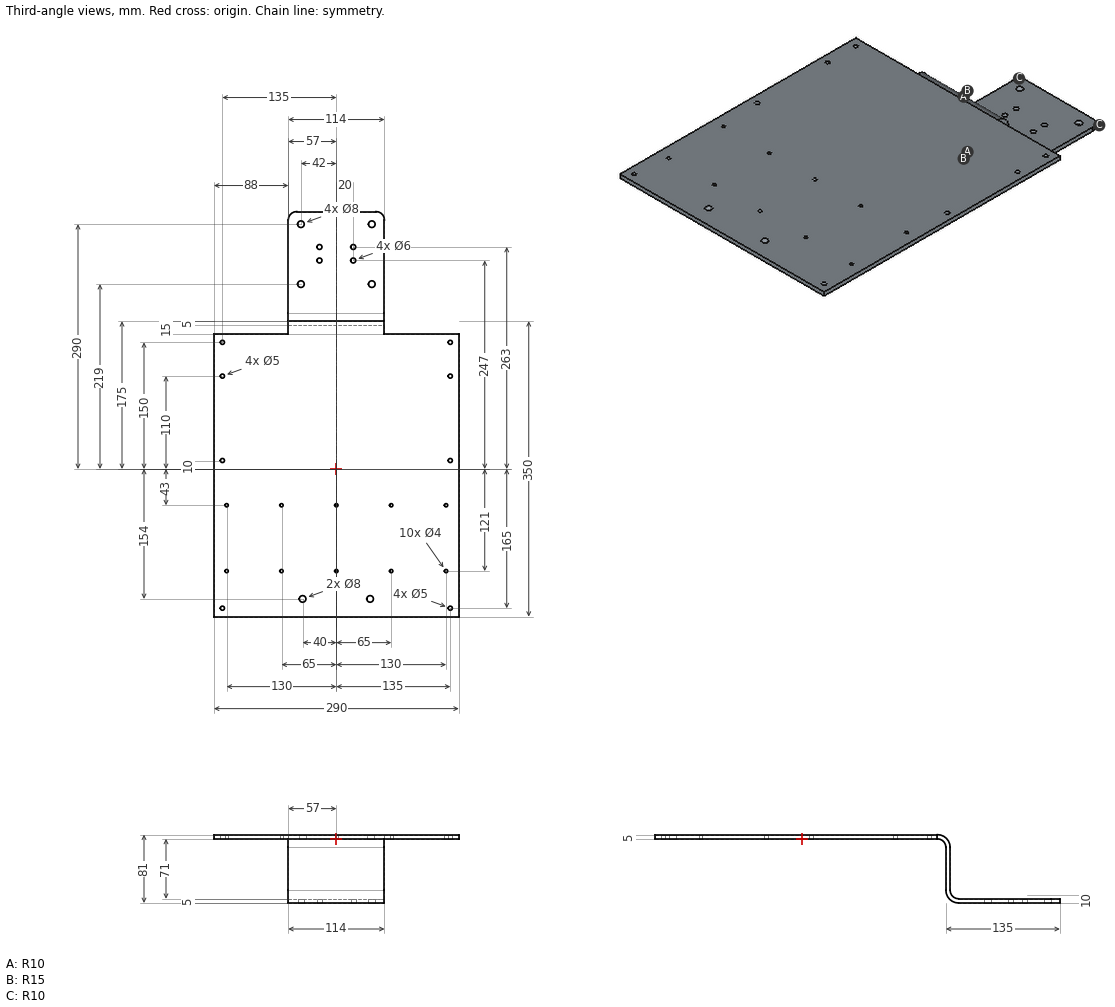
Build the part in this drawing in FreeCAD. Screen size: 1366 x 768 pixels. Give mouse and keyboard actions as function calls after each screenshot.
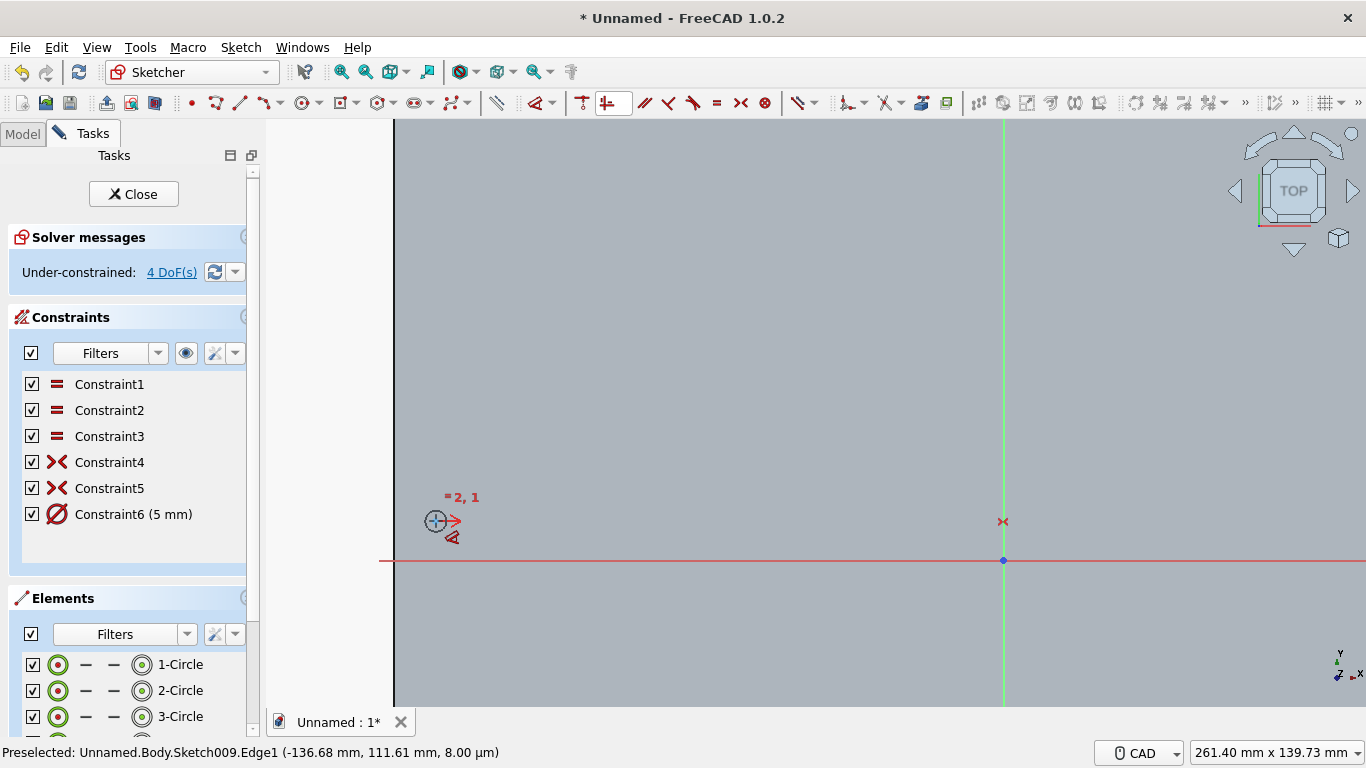
click(436, 521)
click(402, 541)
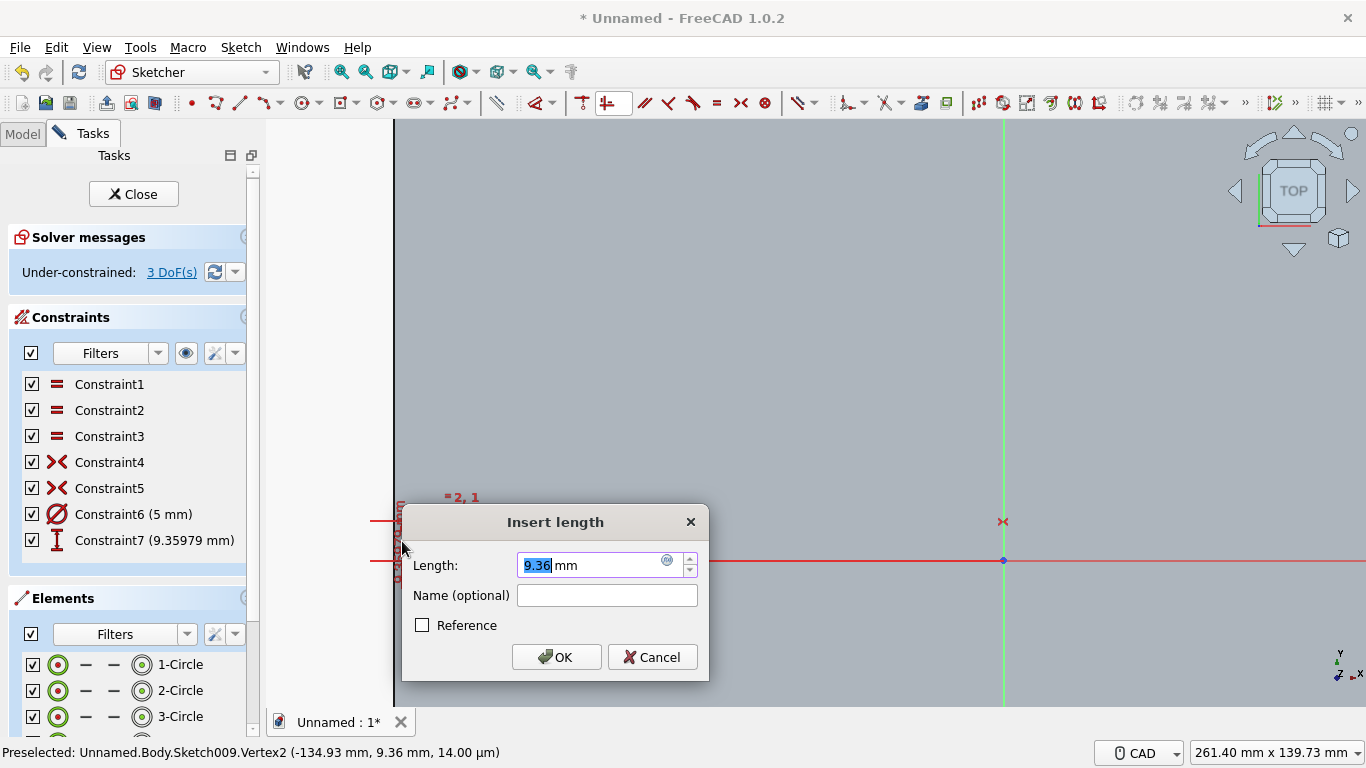
text(10)
key(Return)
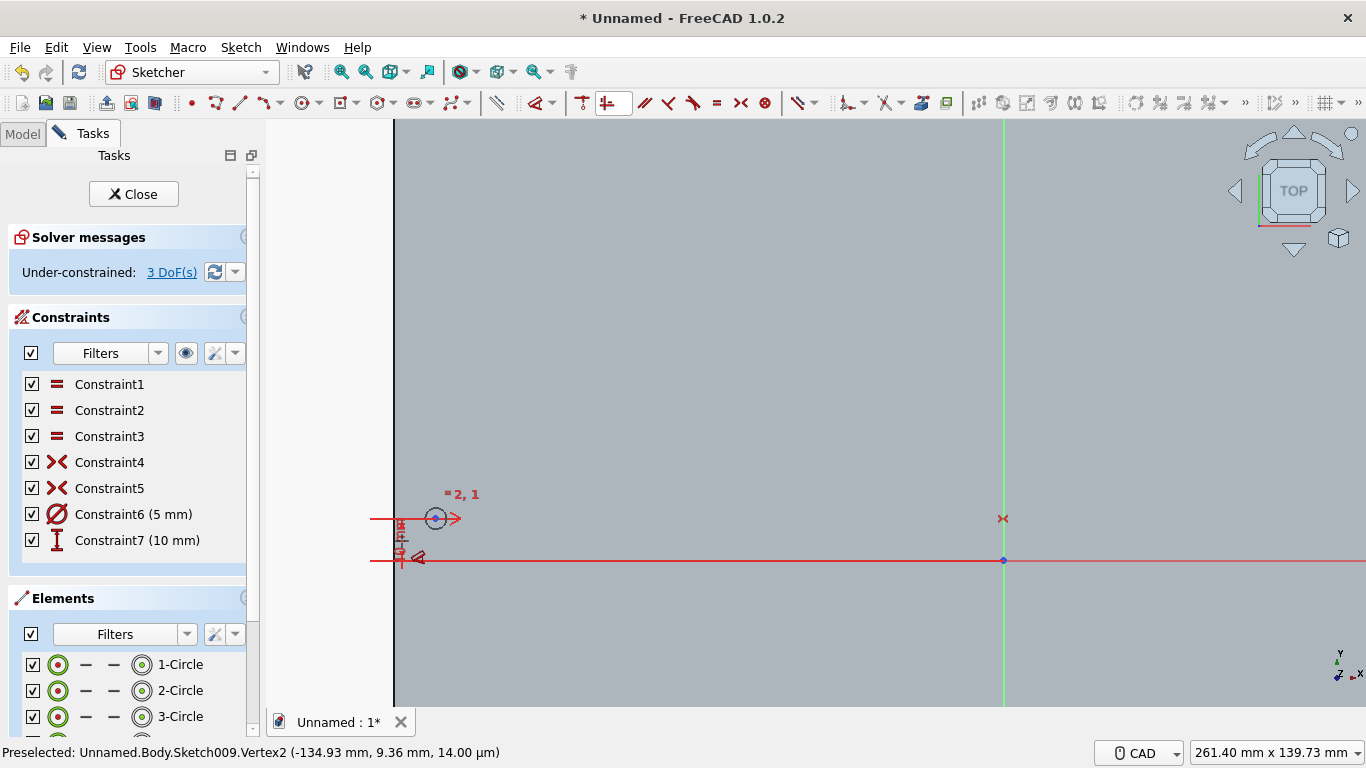
scroll(436, 521, down, 3)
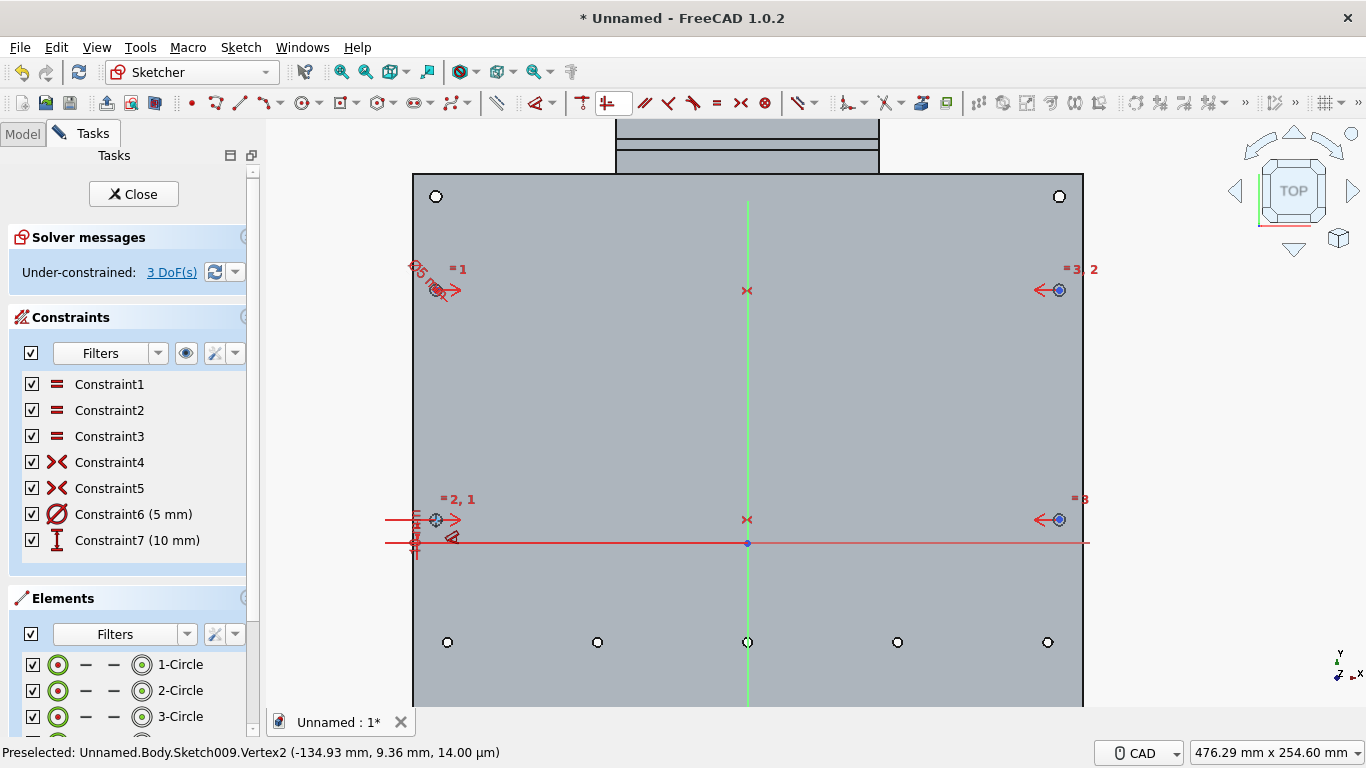
click(436, 290)
click(592, 577)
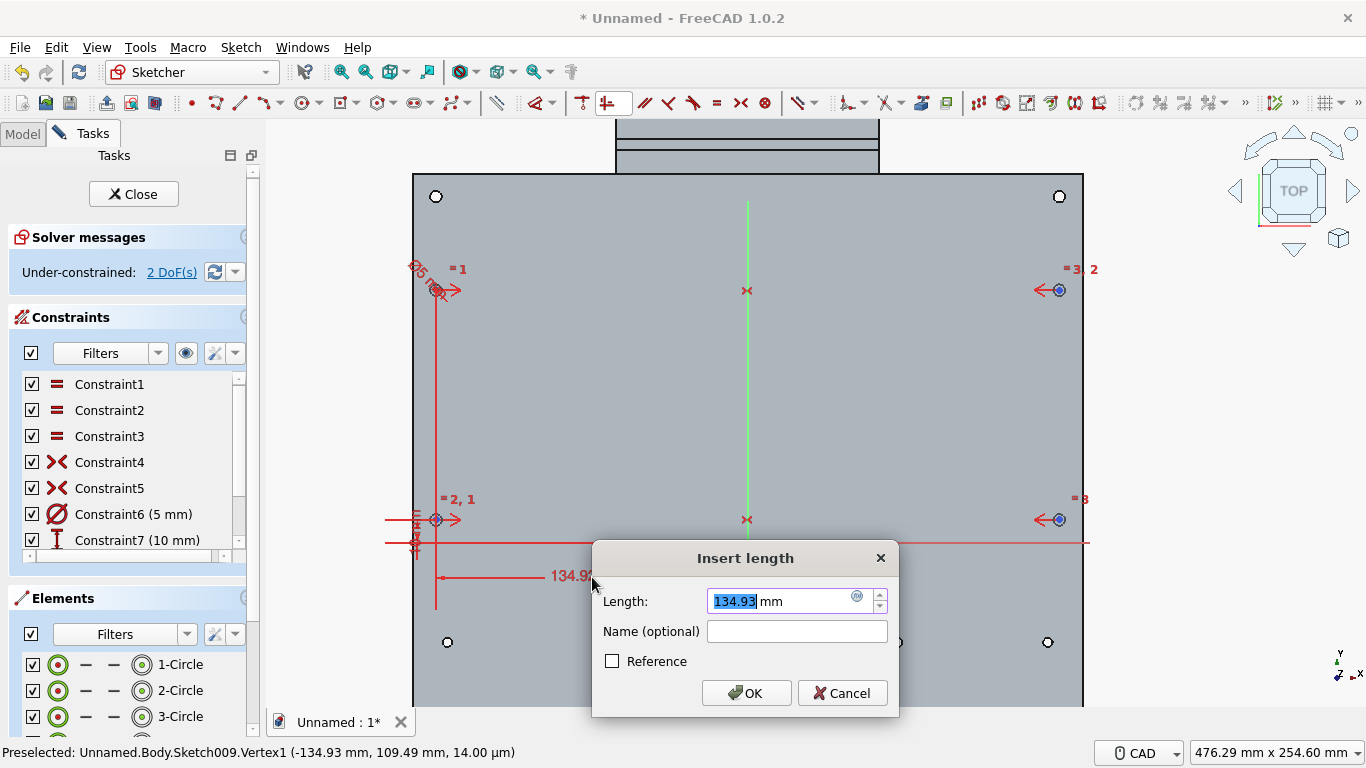
text(135)
key(Return)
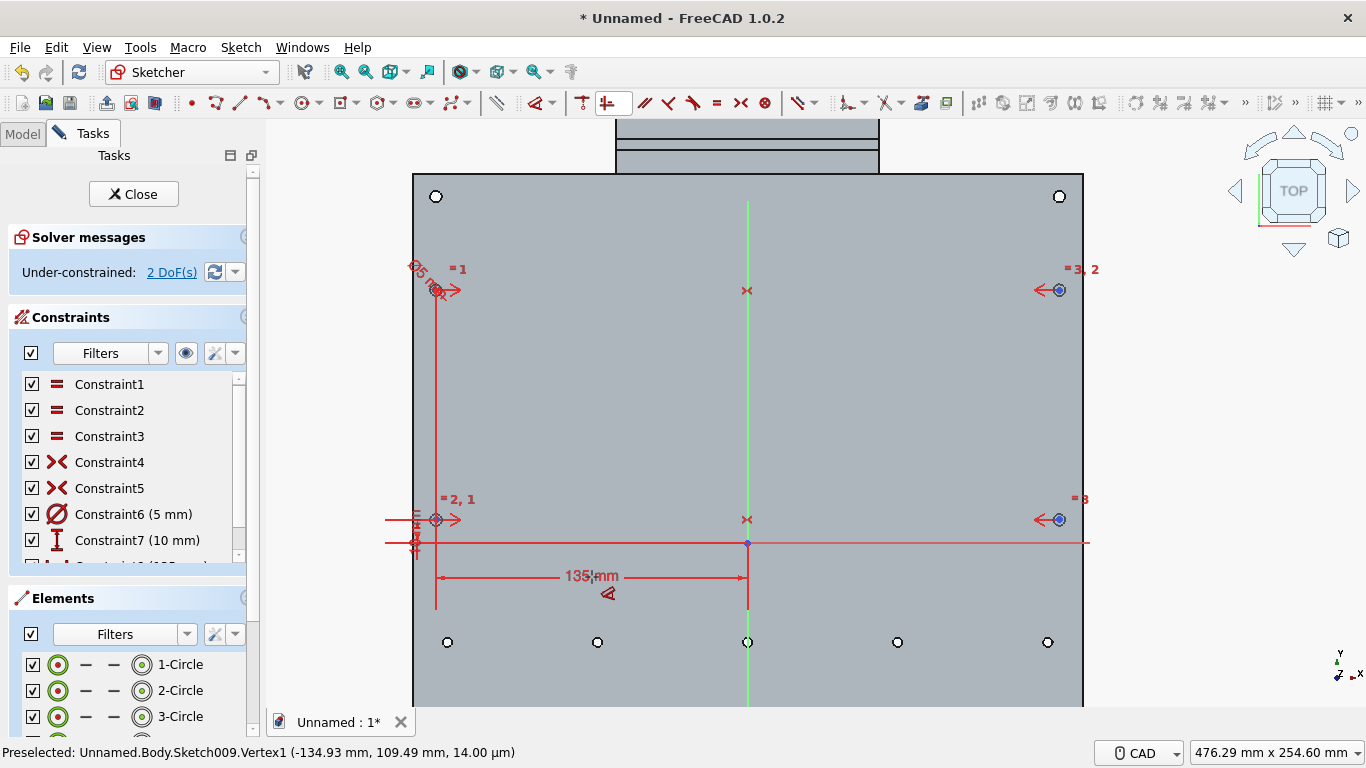
click(436, 290)
click(402, 417)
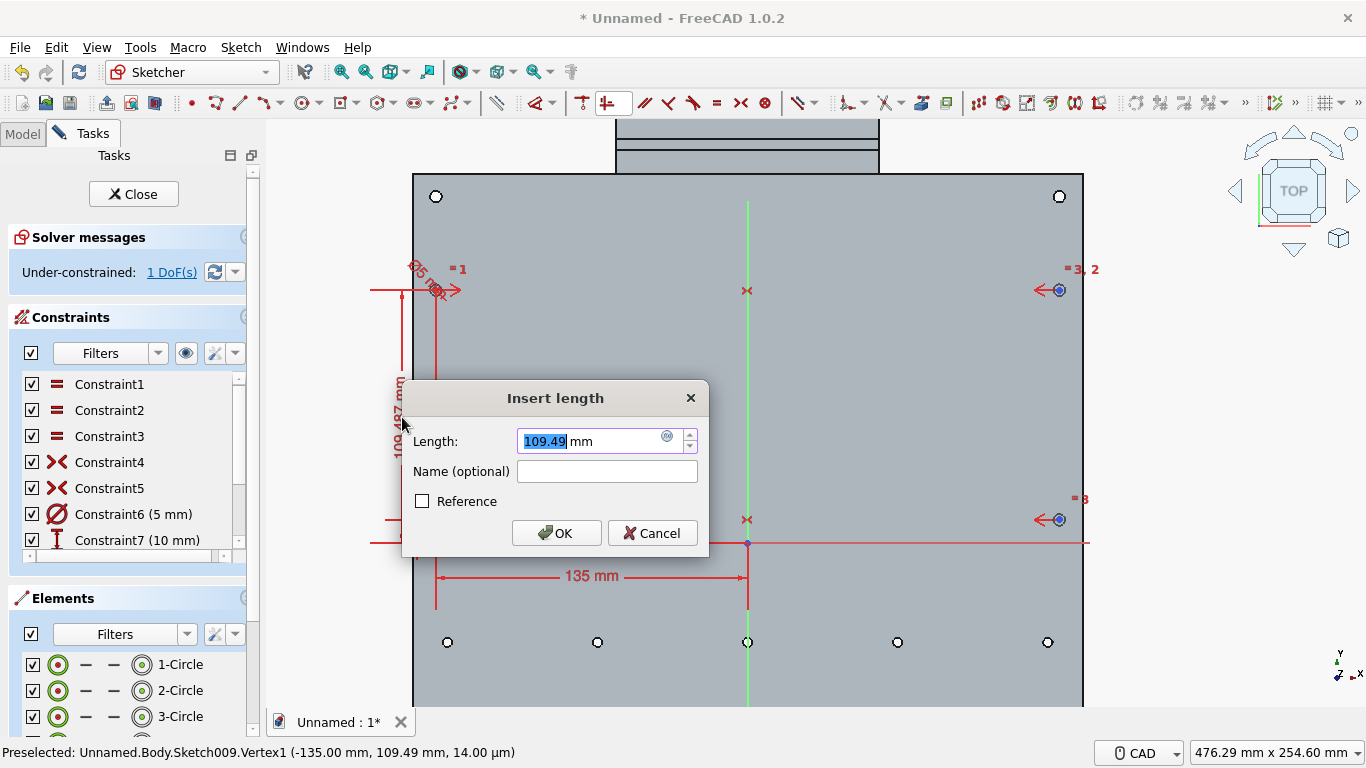
text(110)
key(Return)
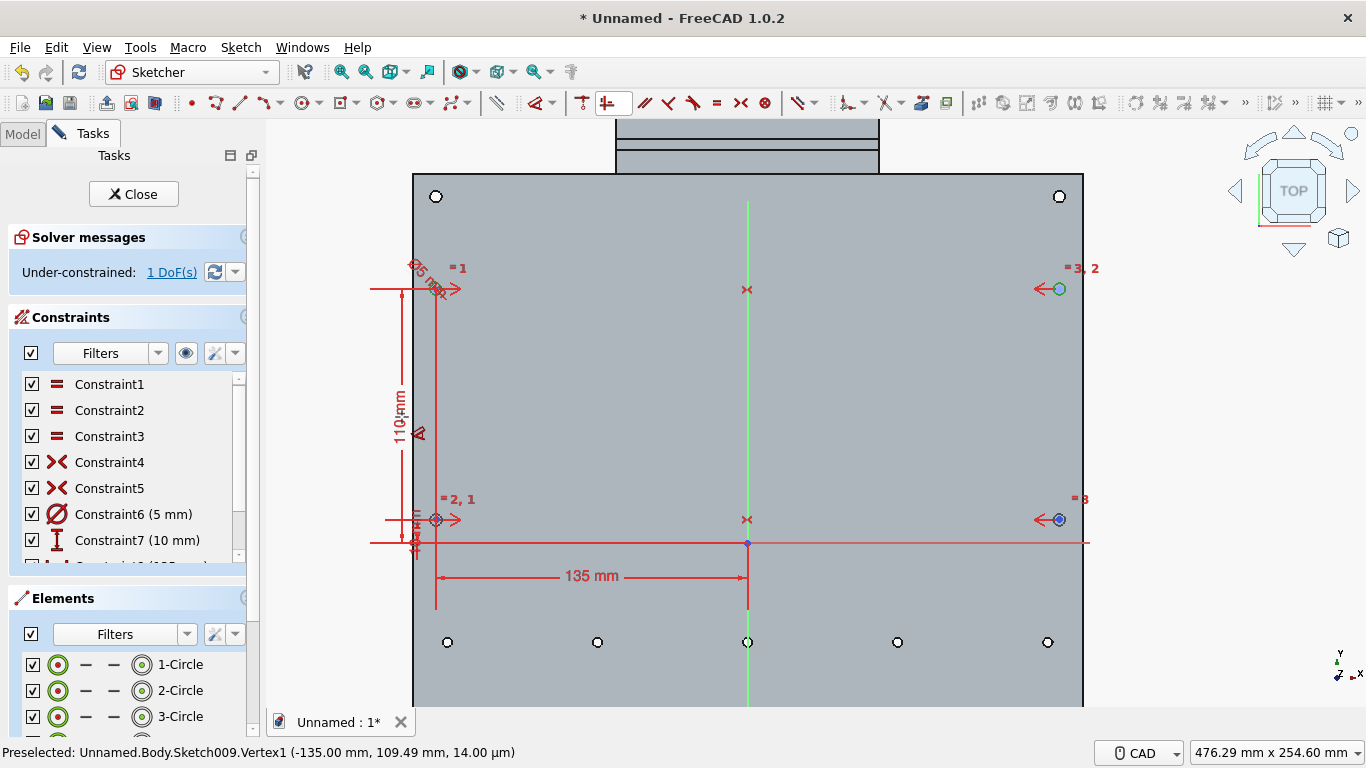
click(436, 520)
click(520, 577)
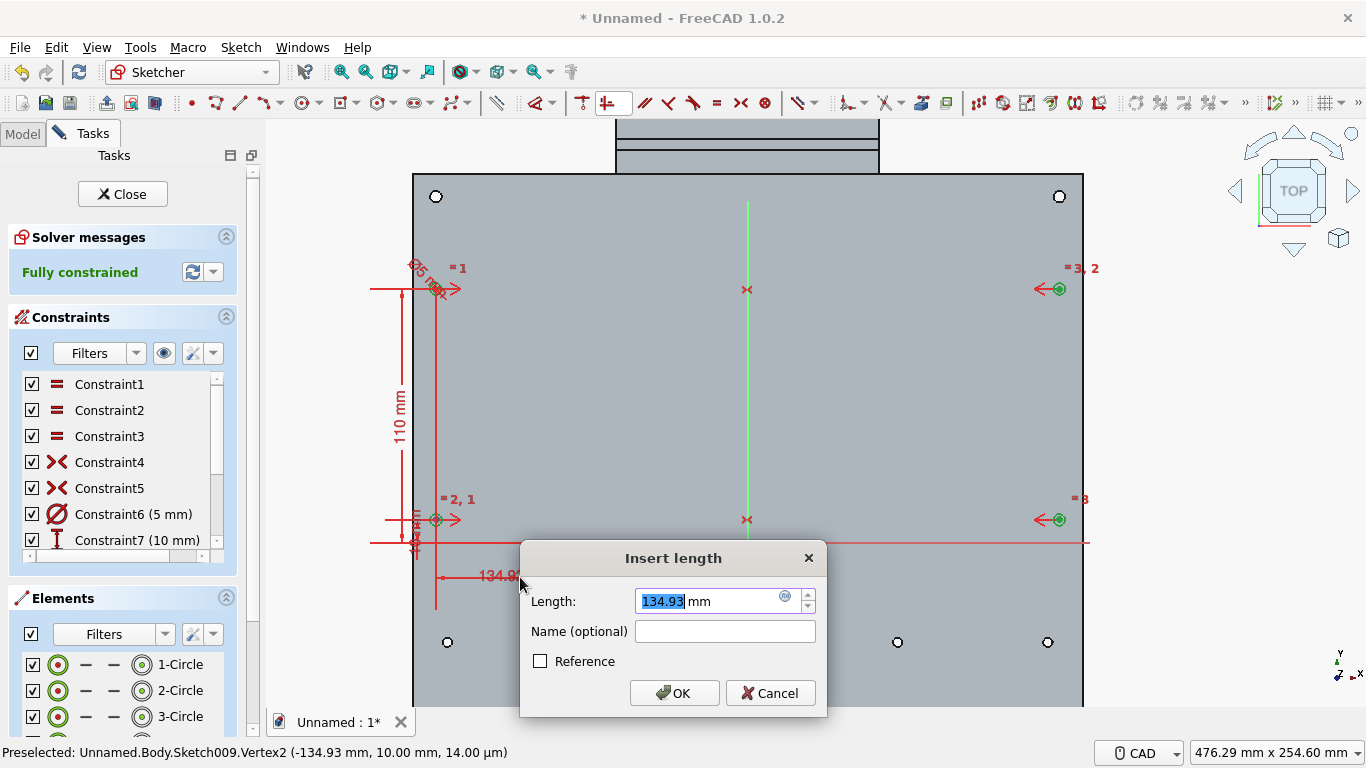
text(135)
key(Return)
key(Escape)